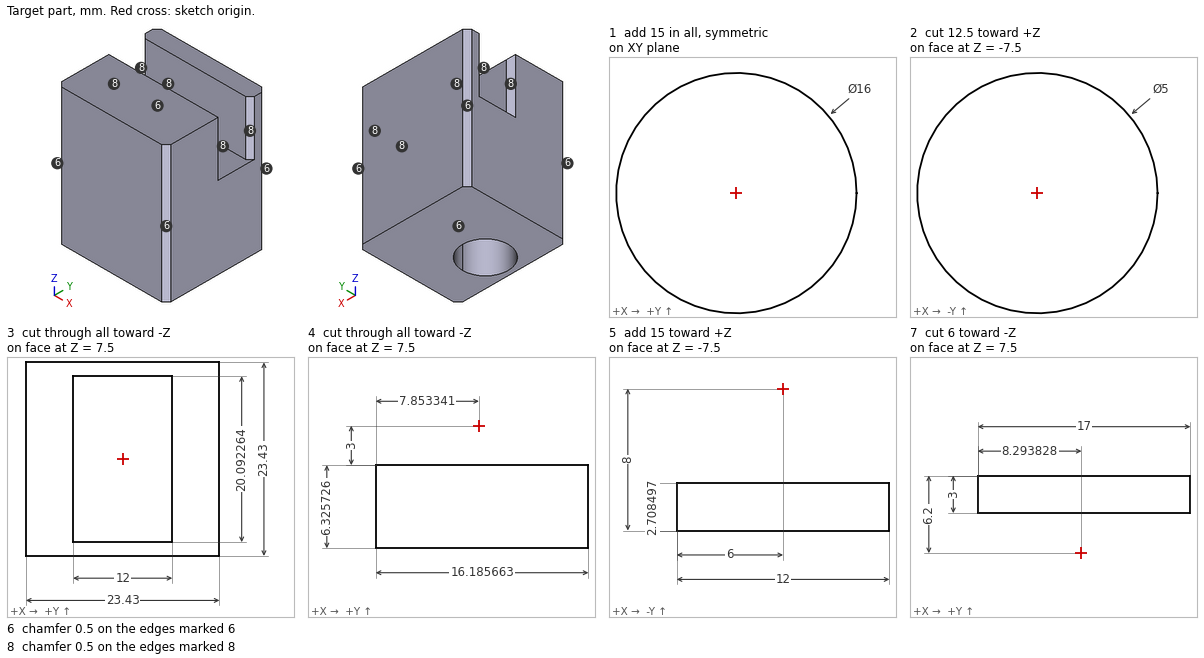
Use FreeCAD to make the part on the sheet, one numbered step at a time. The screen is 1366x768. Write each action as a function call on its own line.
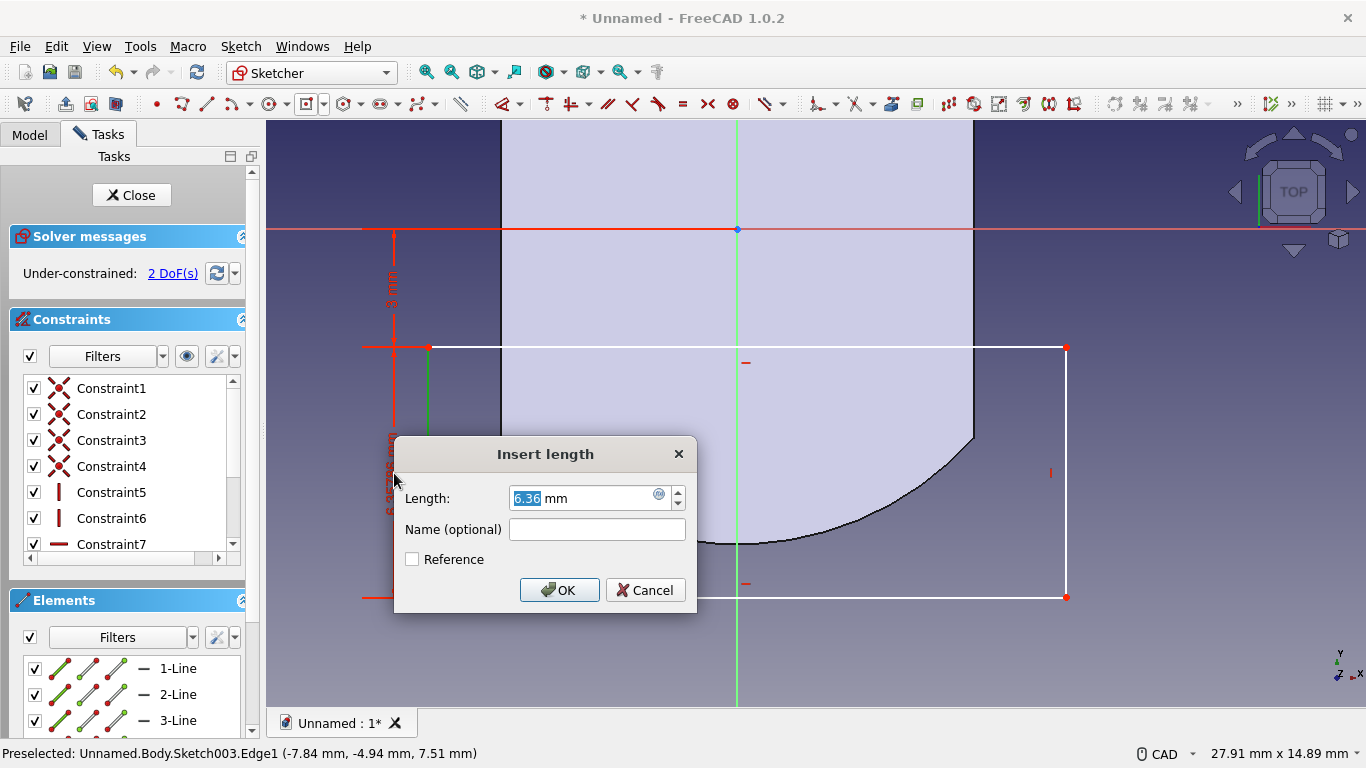
text(6.325726)
key(Return)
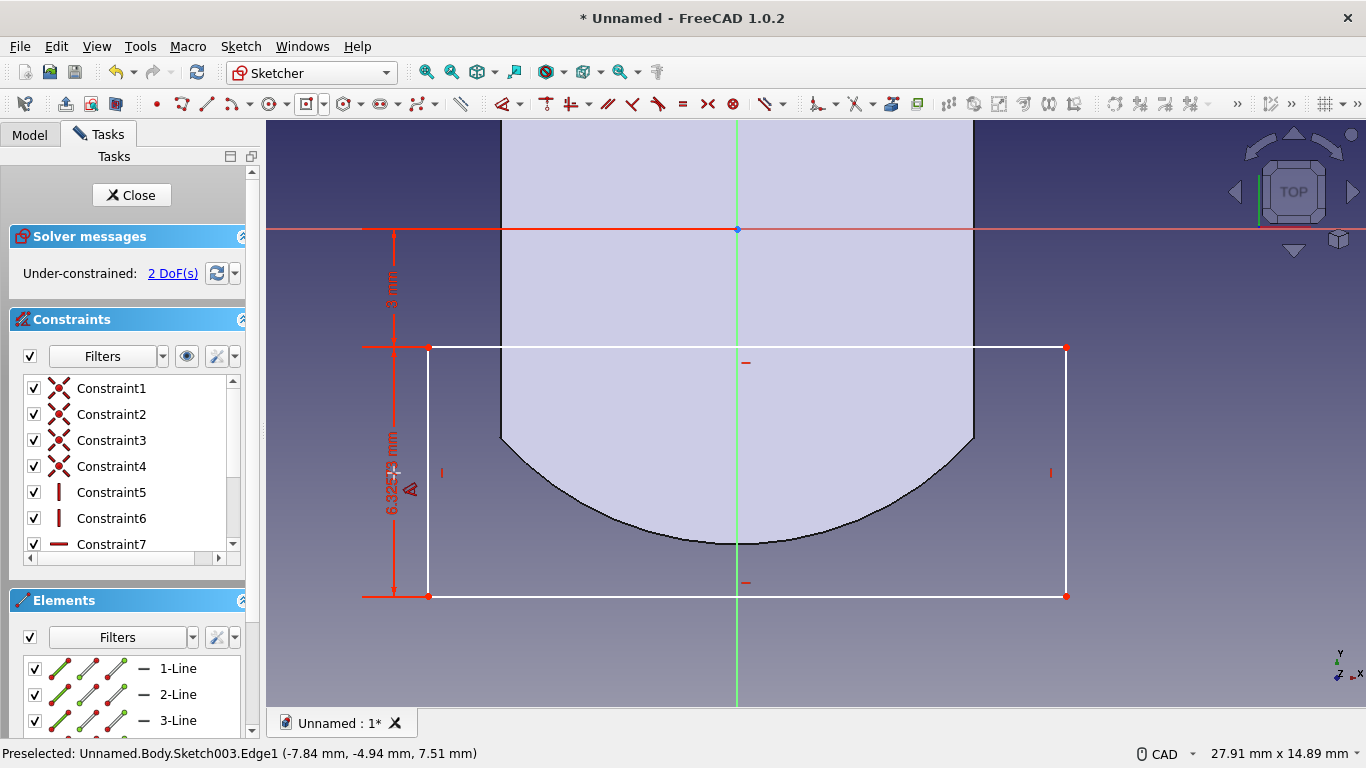
click(619, 597)
click(600, 631)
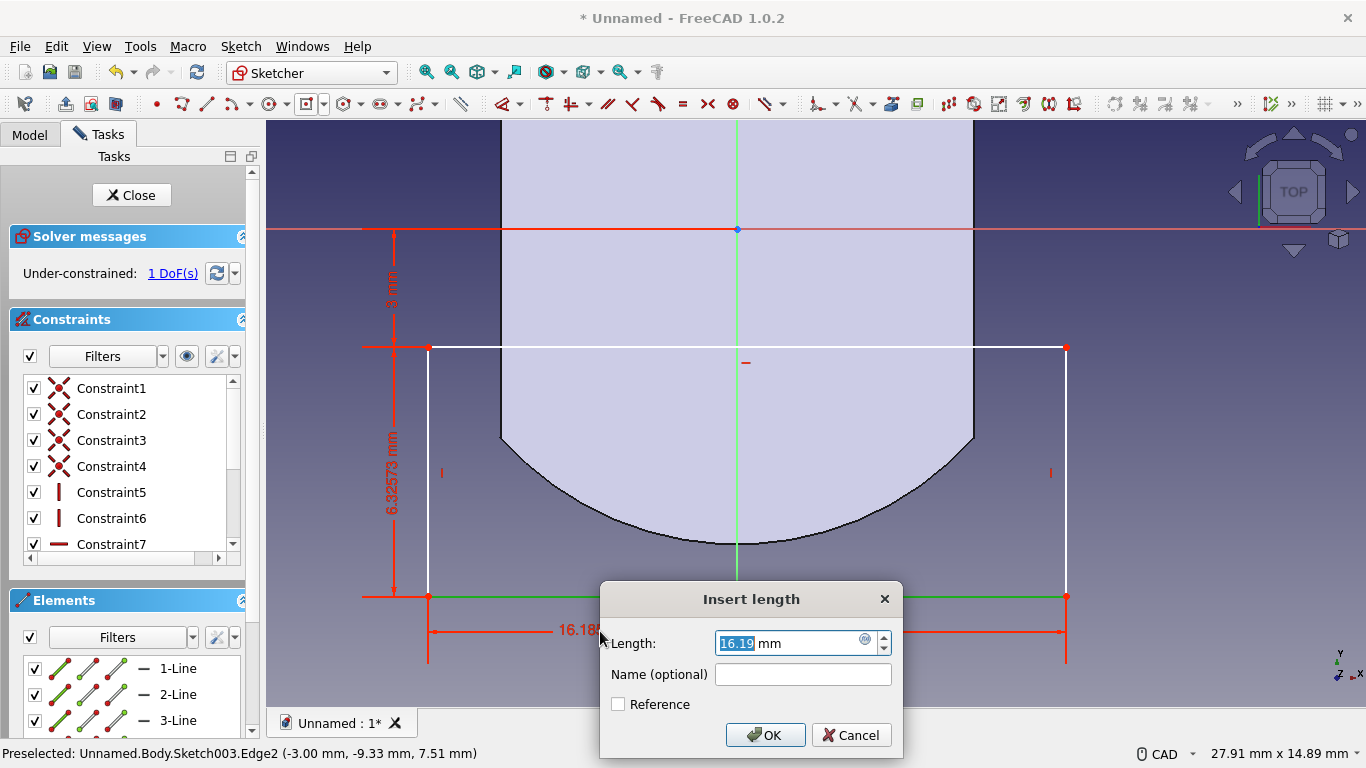
text(16.185663)
key(Return)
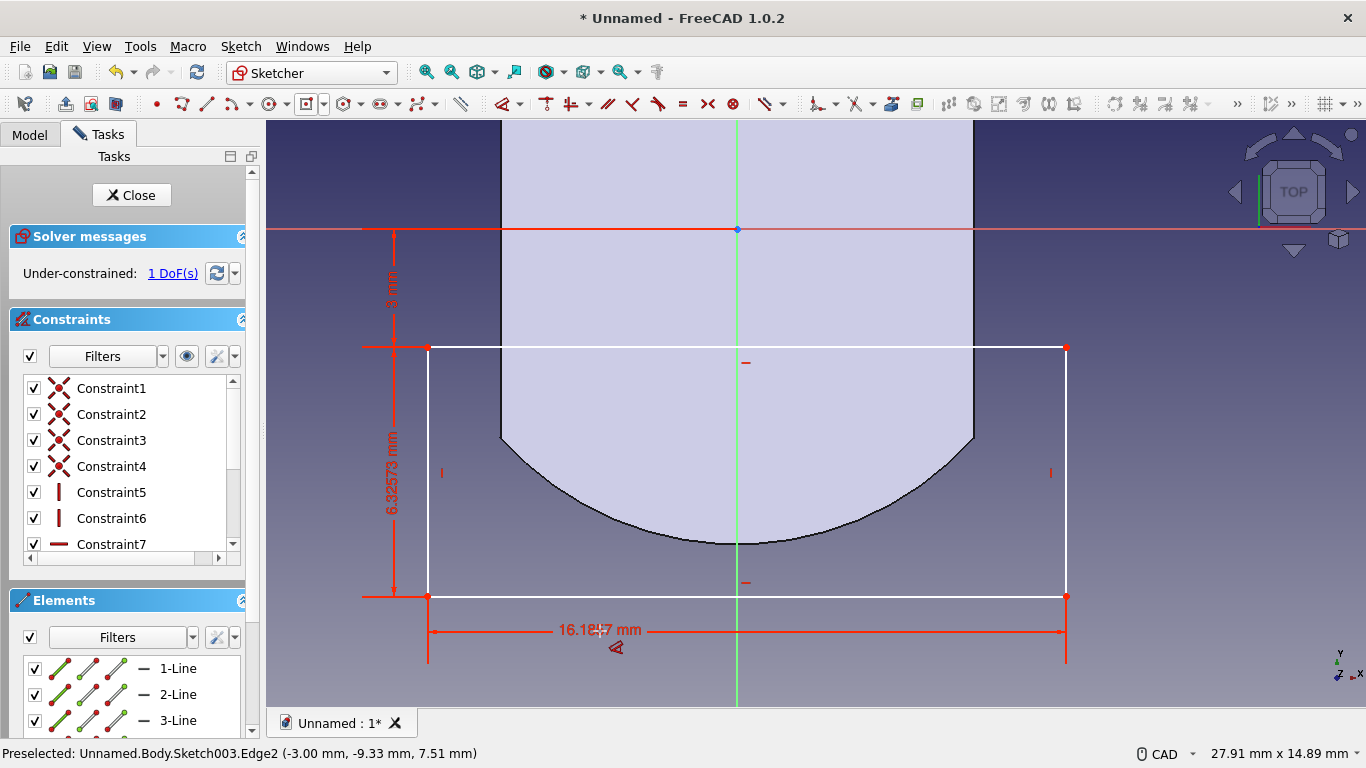
click(428, 347)
click(583, 195)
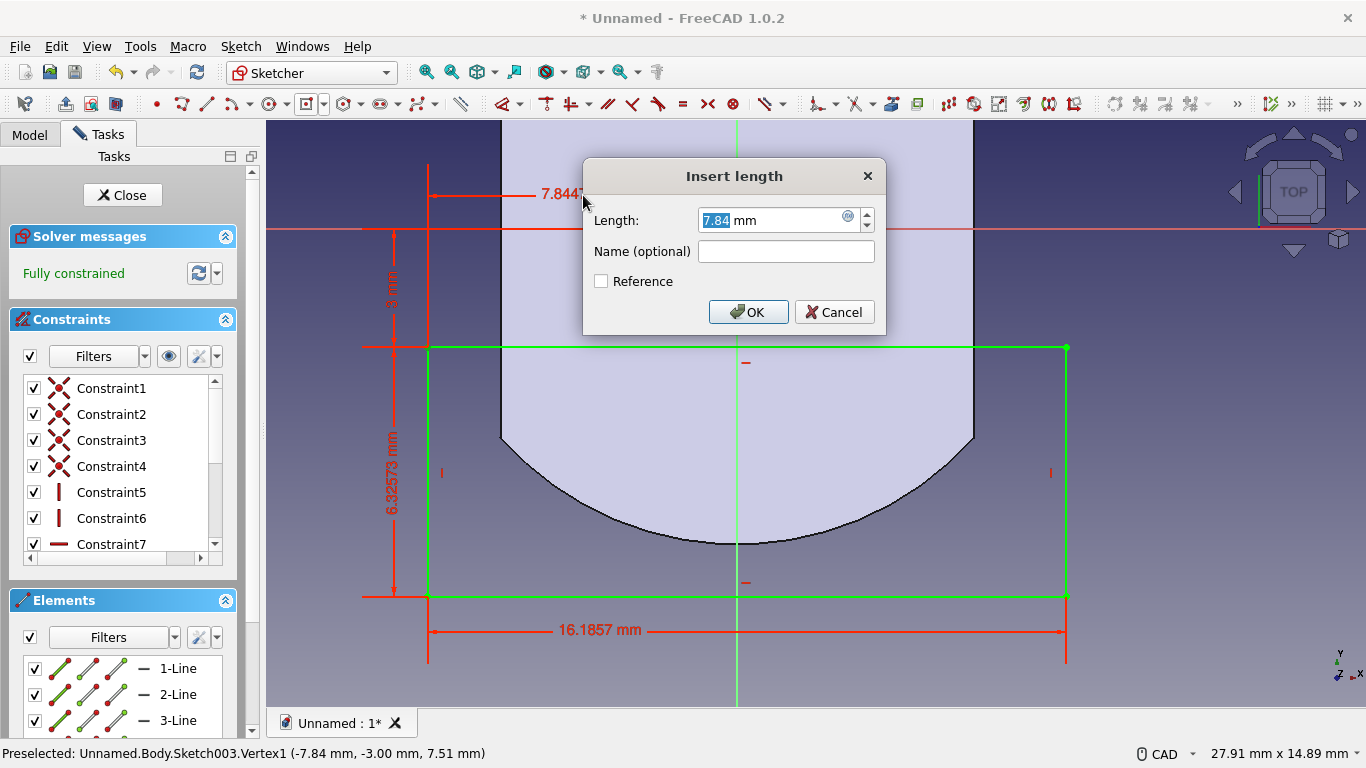
text(7.853341)
key(Return)
key(Escape)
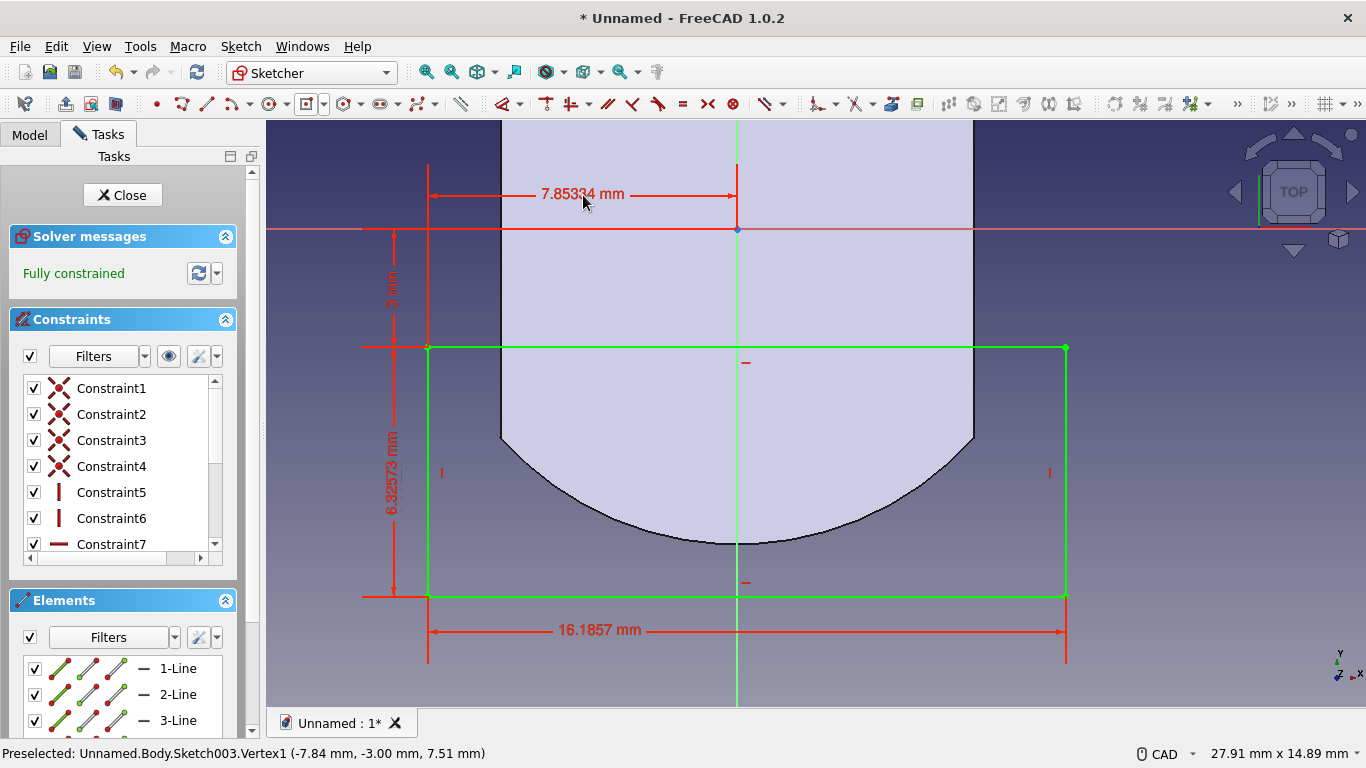
click(123, 195)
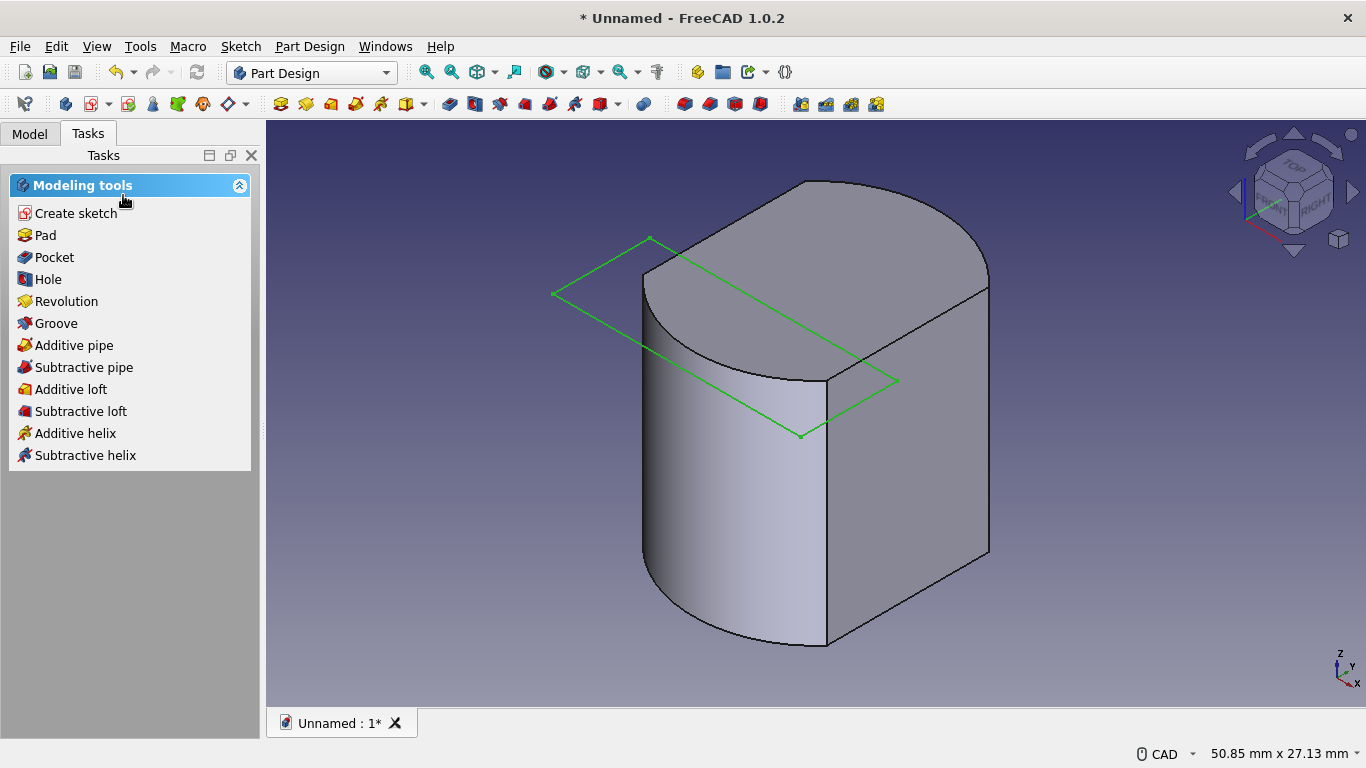
click(450, 104)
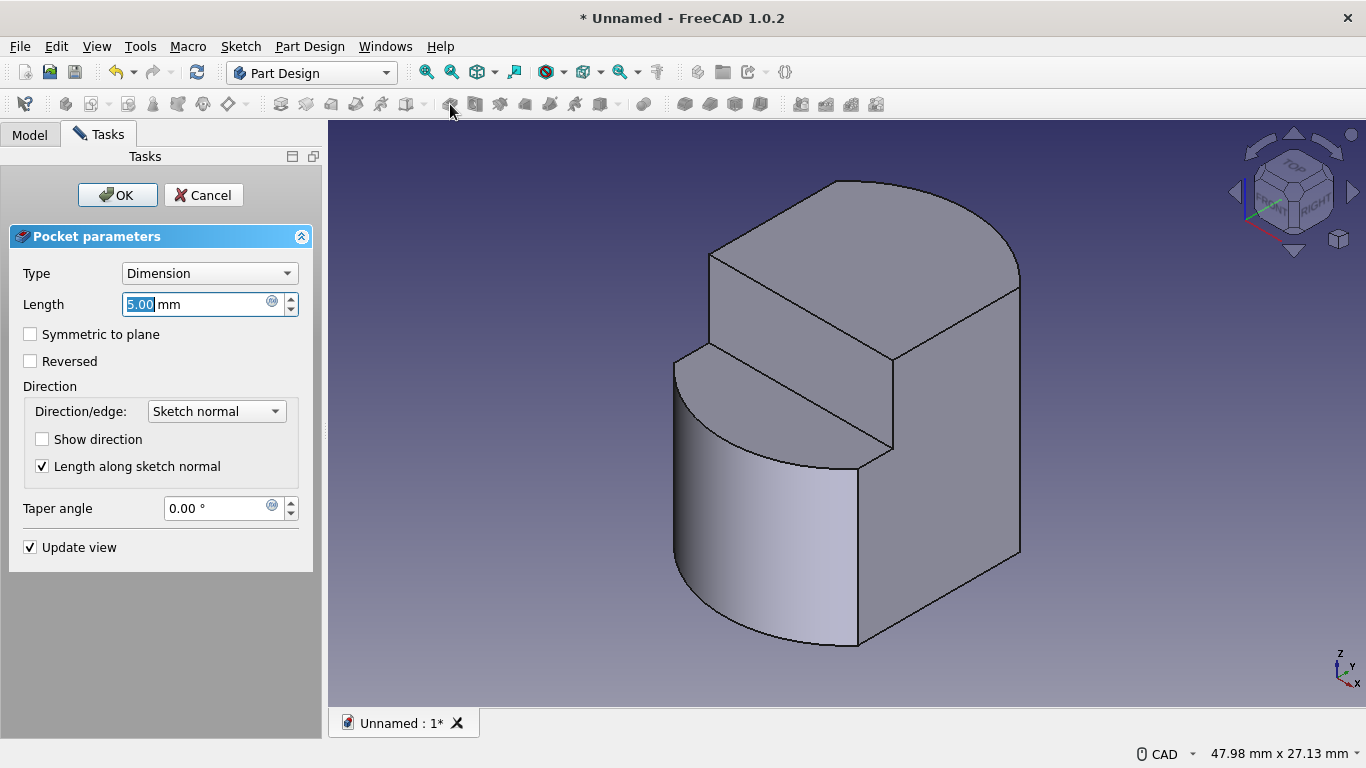
click(210, 274)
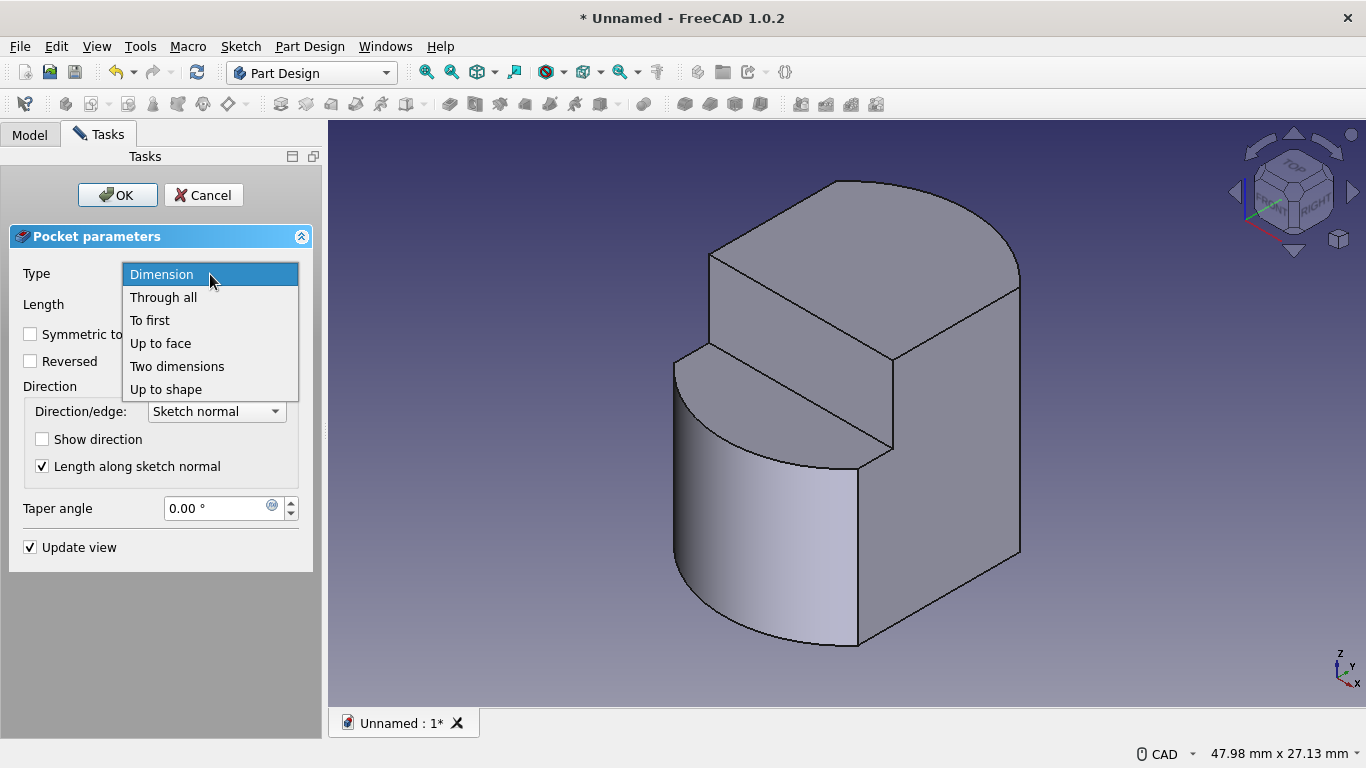
click(208, 298)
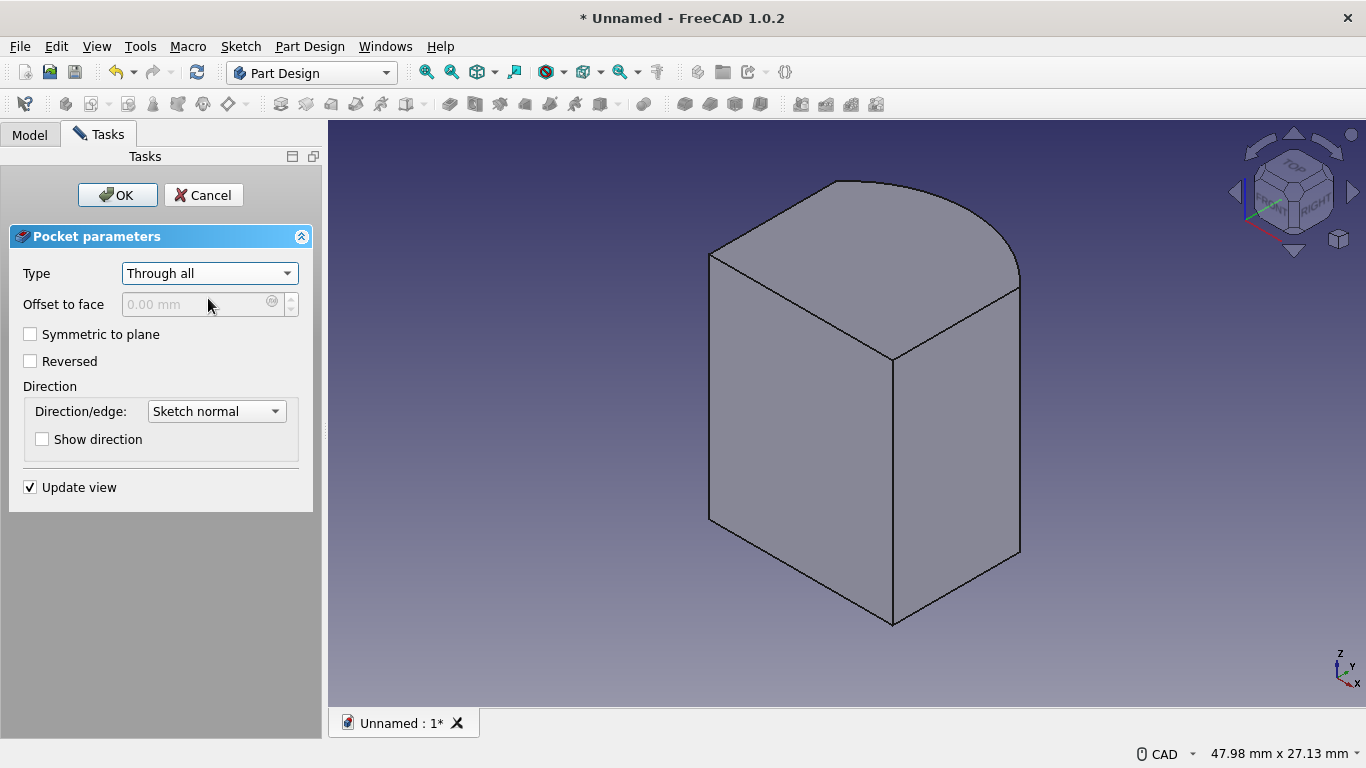
click(118, 195)